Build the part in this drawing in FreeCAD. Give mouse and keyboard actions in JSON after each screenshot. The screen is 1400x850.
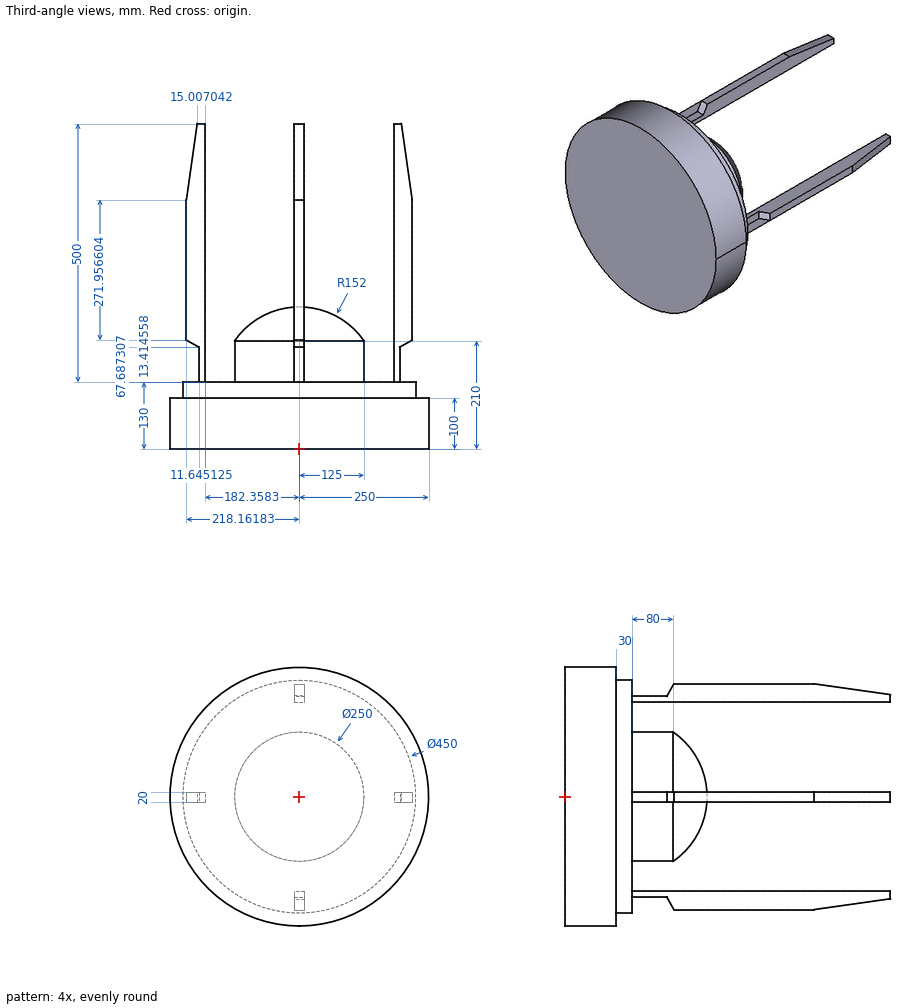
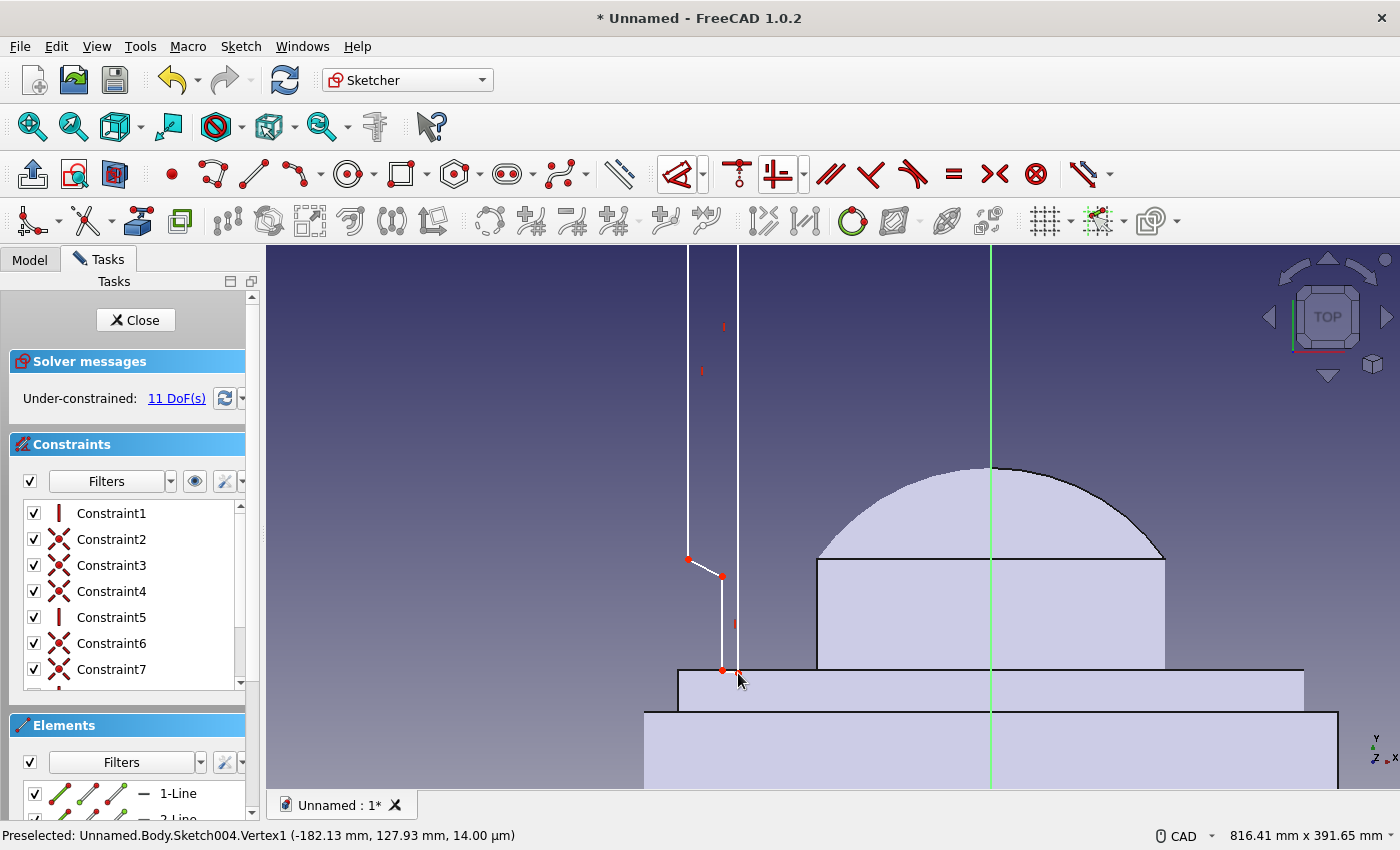
{"action": "scroll", "coordinate": [721, 577], "scroll_direction": "down", "scroll_amount": 5}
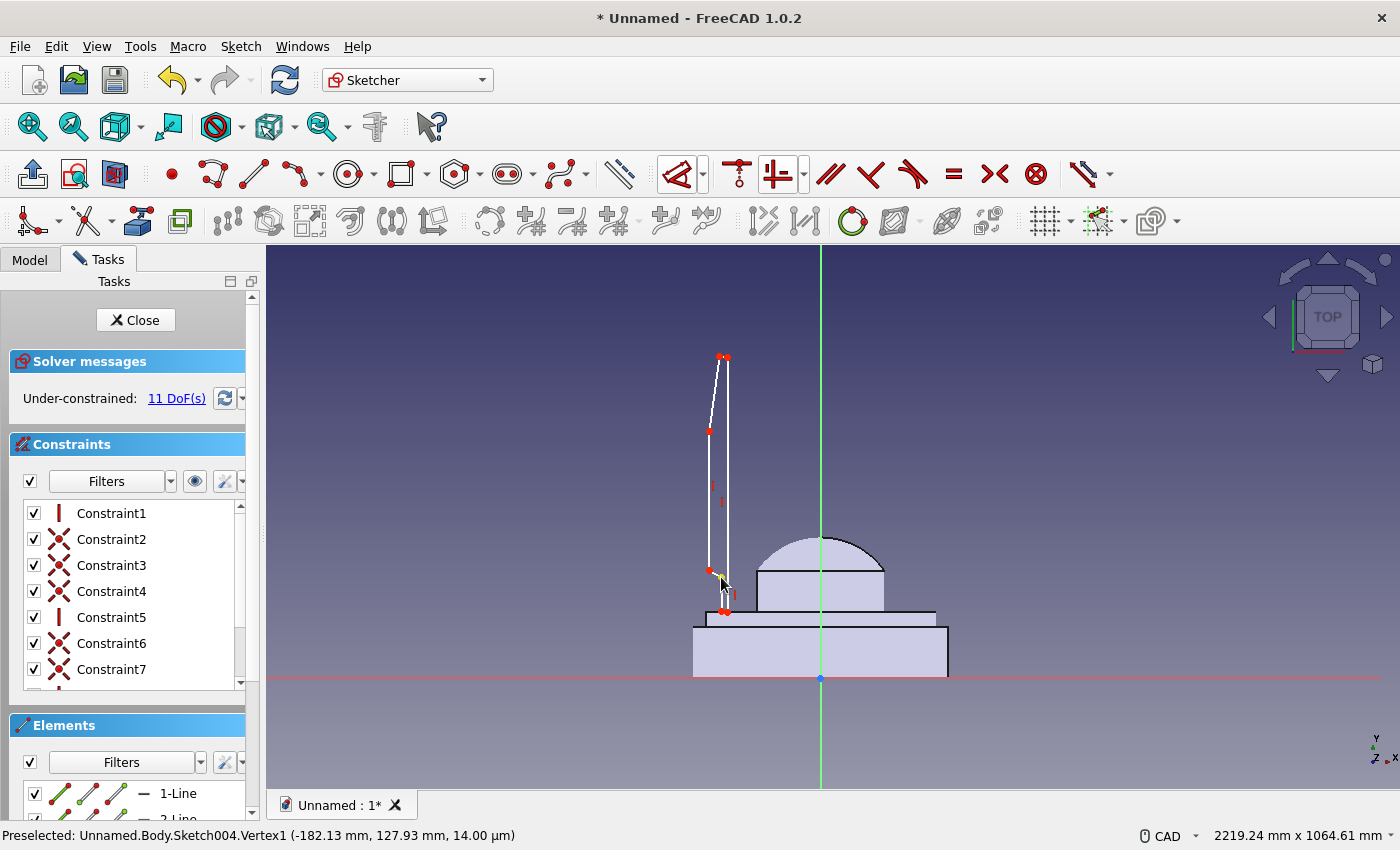
{"action": "scroll", "coordinate": [724, 357], "scroll_direction": "up", "scroll_amount": 7}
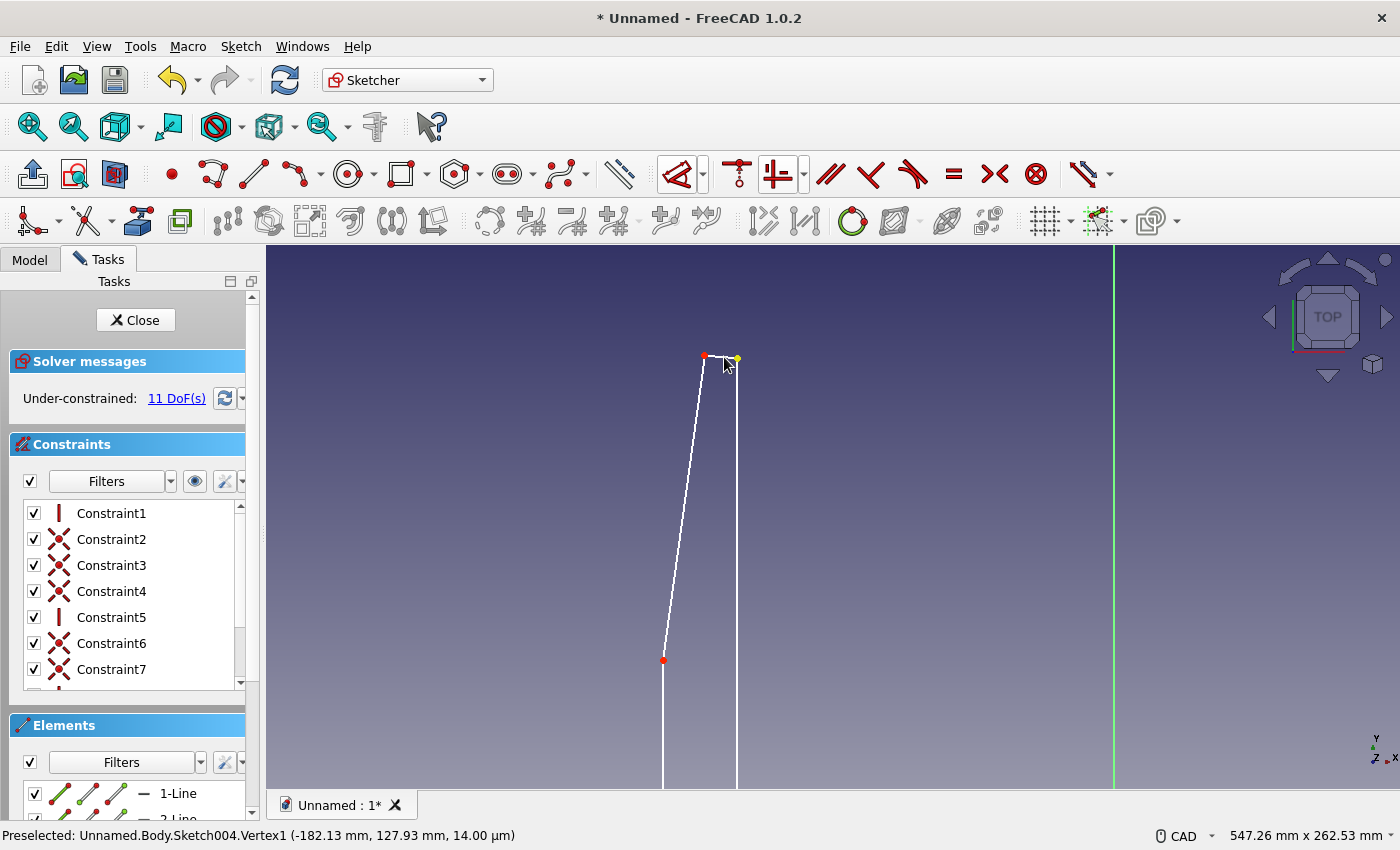
{"action": "left_click", "coordinate": [721, 357]}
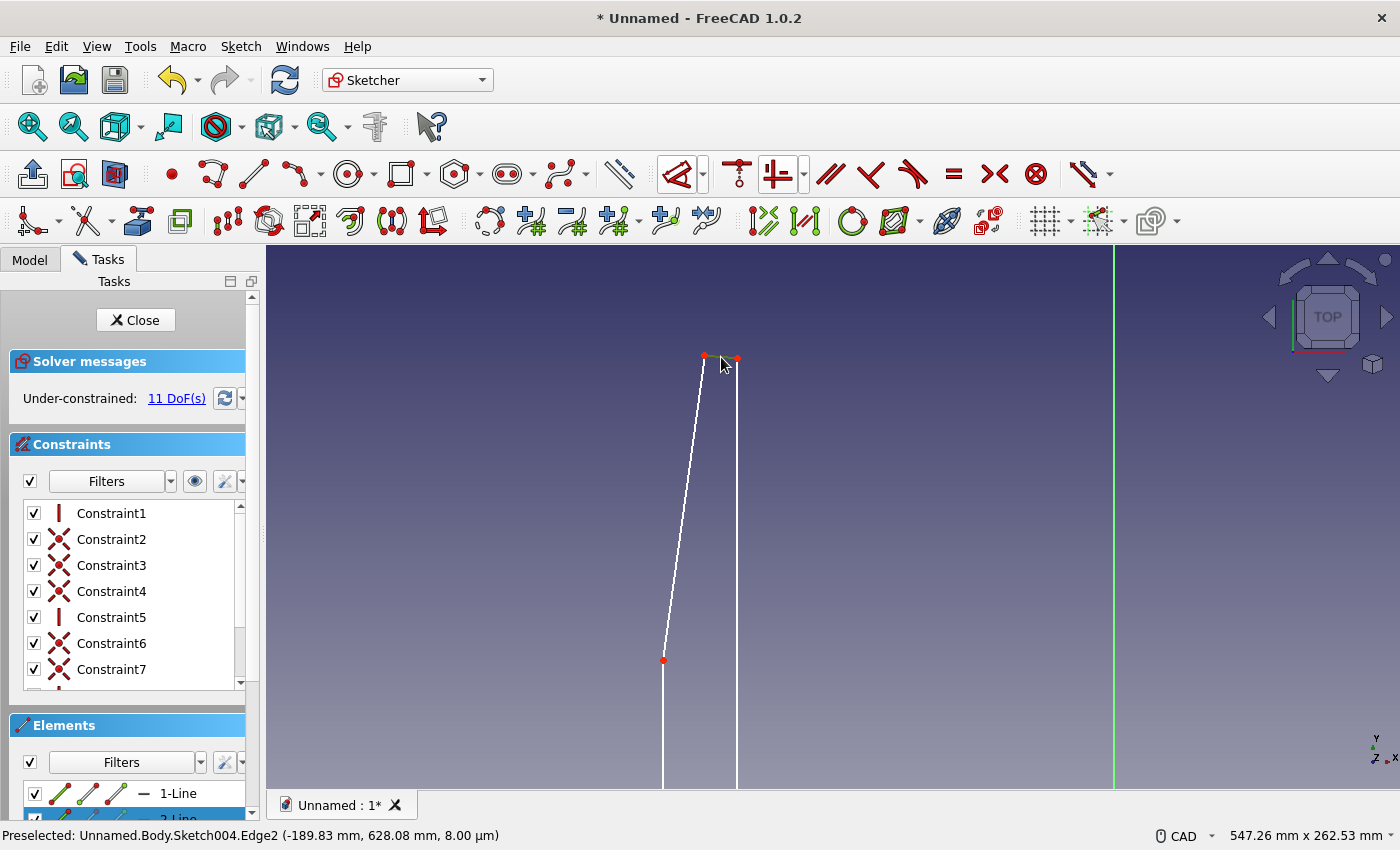
{"action": "left_click", "coordinate": [804, 174]}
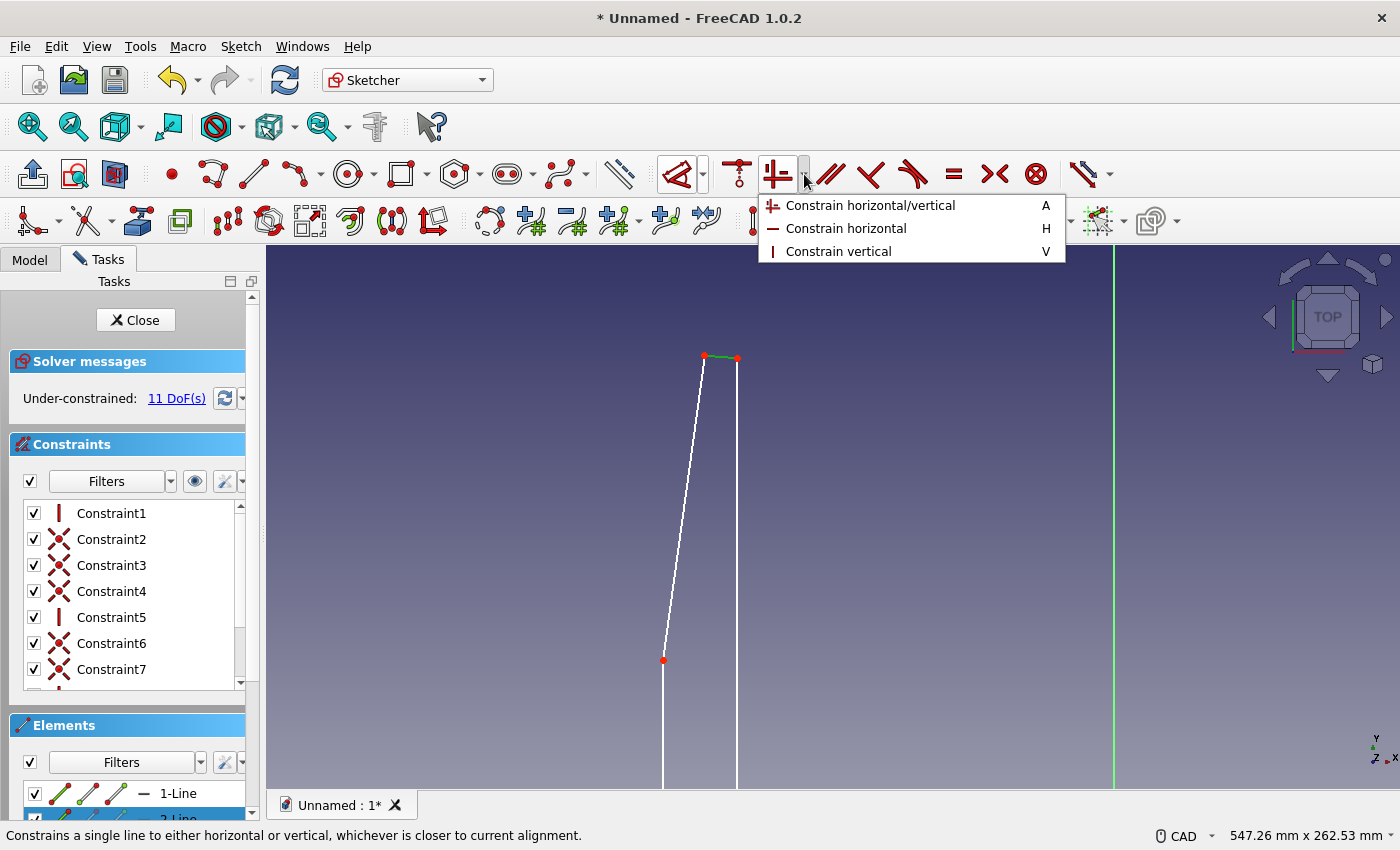
{"action": "left_click", "coordinate": [912, 228]}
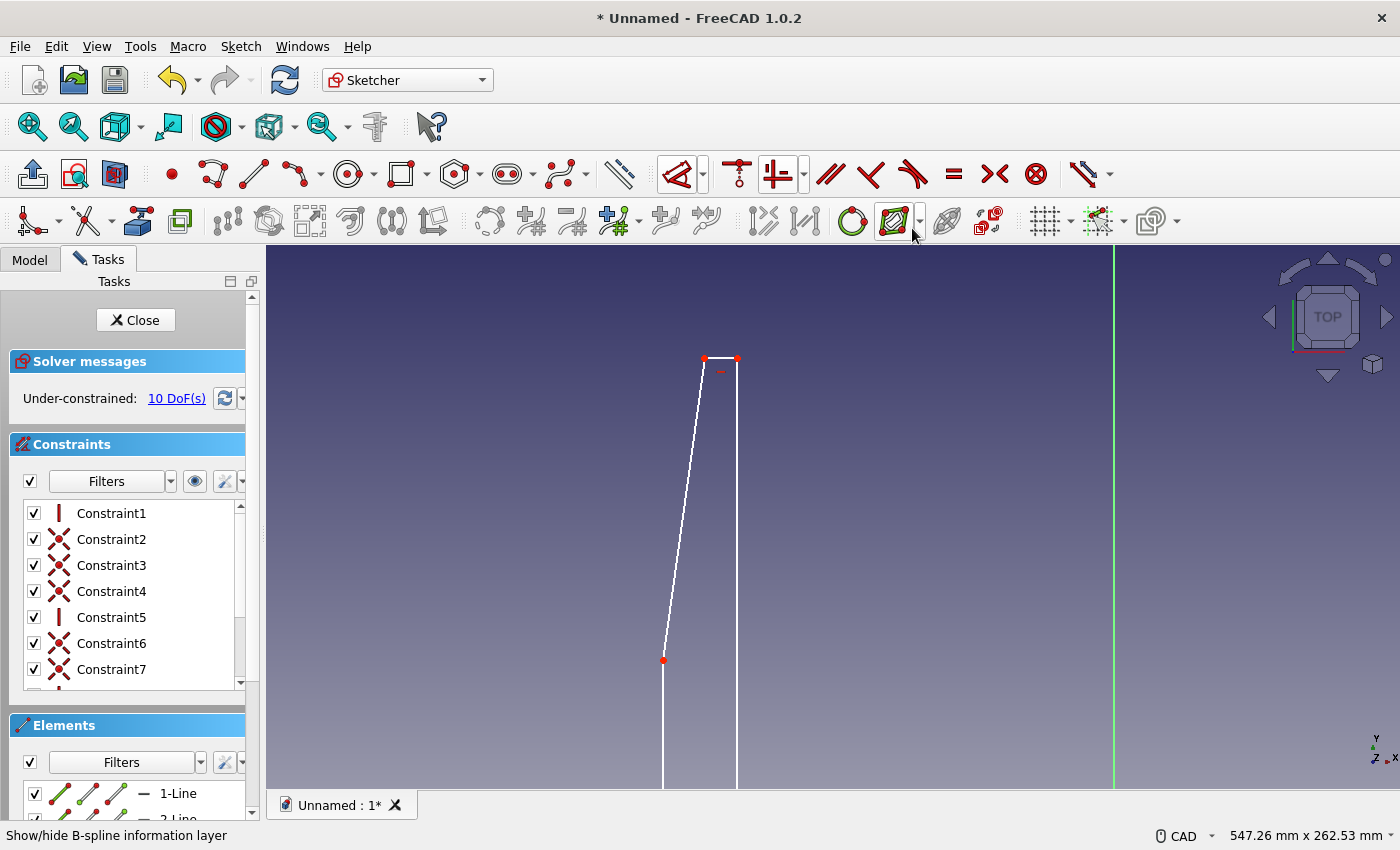
{"action": "scroll", "coordinate": [724, 357], "scroll_direction": "down", "scroll_amount": 7}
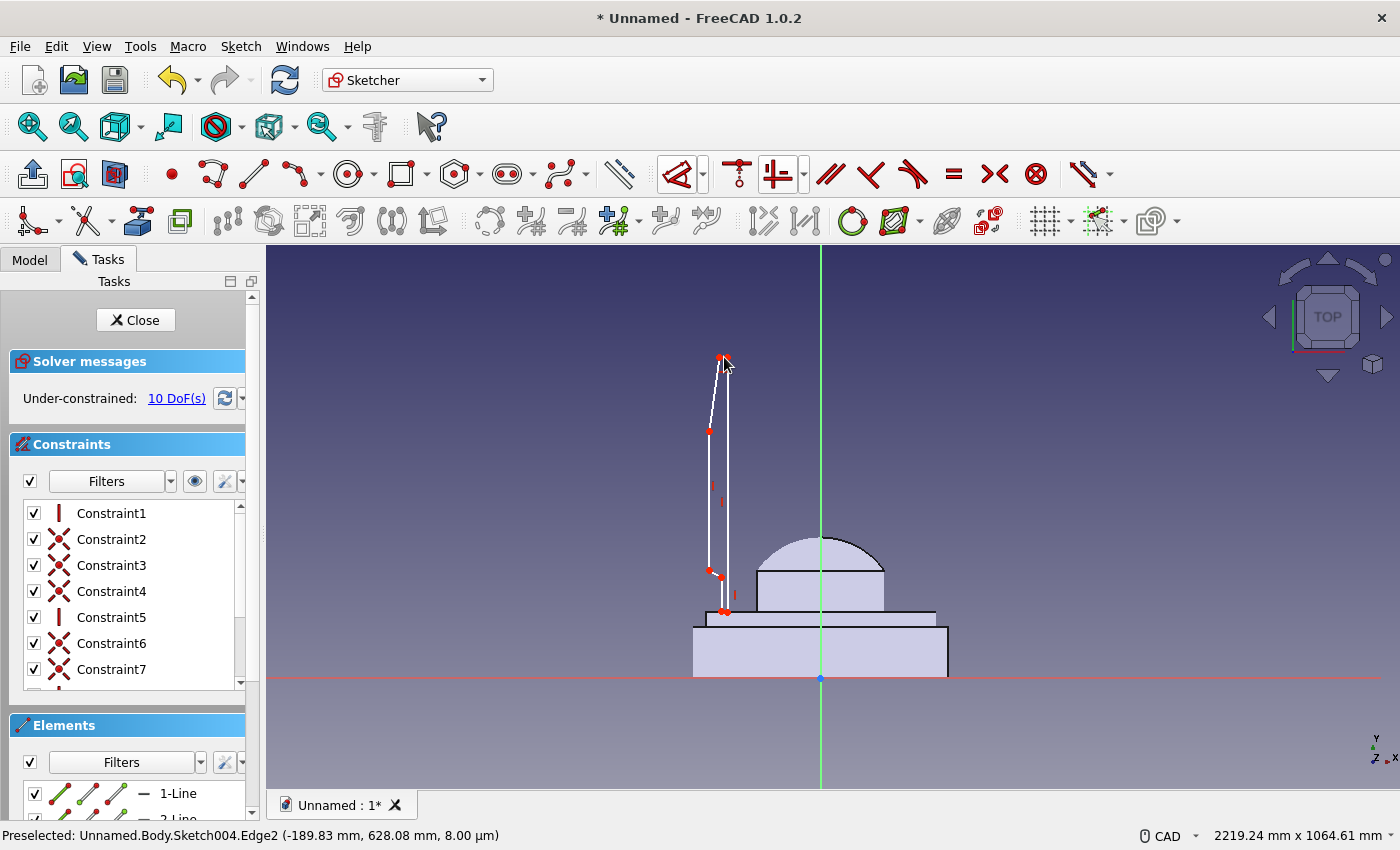
{"action": "scroll", "coordinate": [724, 612], "scroll_direction": "up", "scroll_amount": 9}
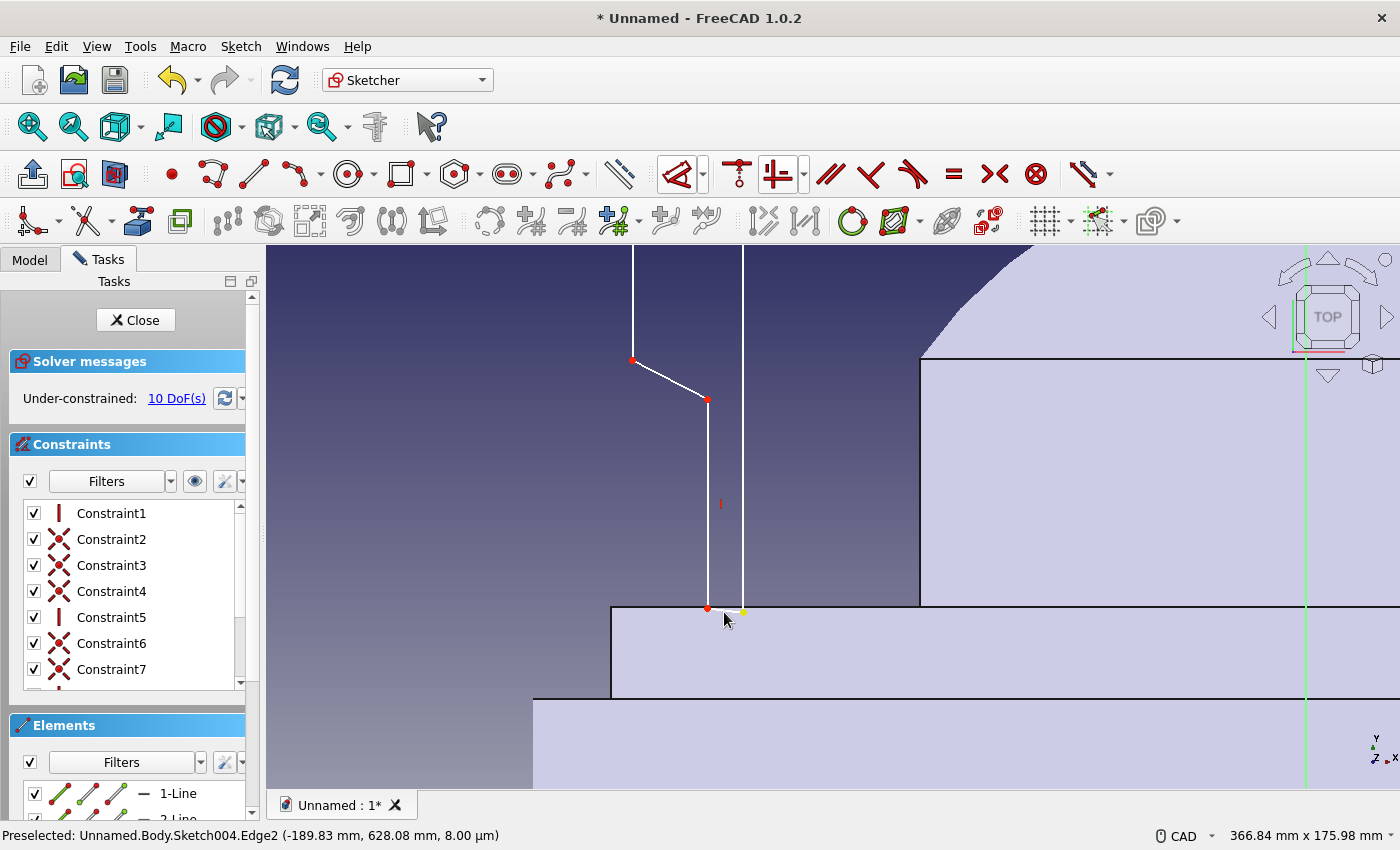
{"action": "left_click", "coordinate": [722, 610]}